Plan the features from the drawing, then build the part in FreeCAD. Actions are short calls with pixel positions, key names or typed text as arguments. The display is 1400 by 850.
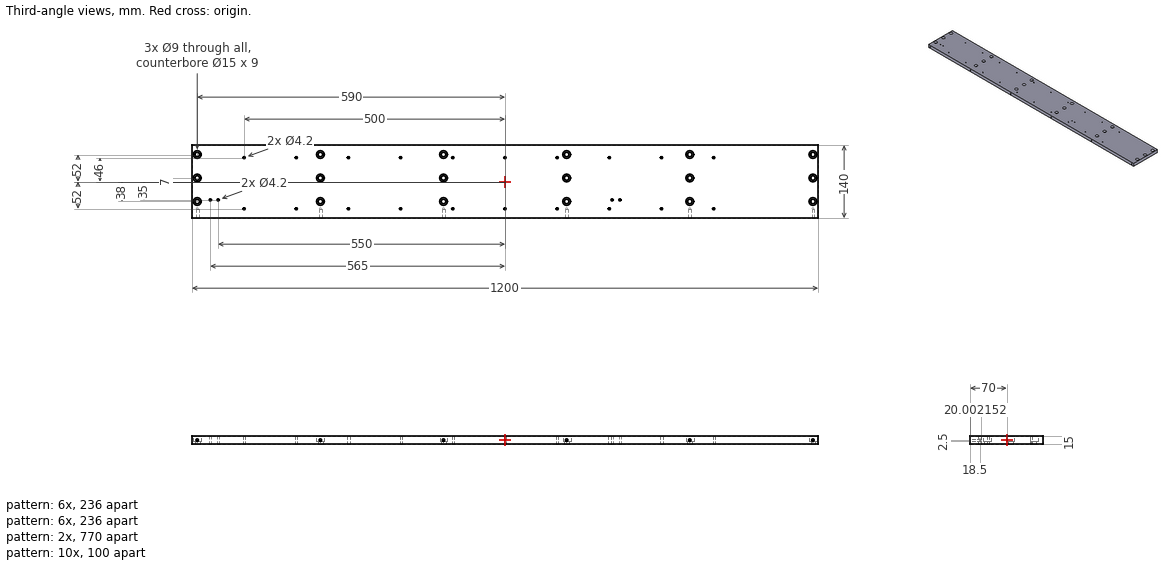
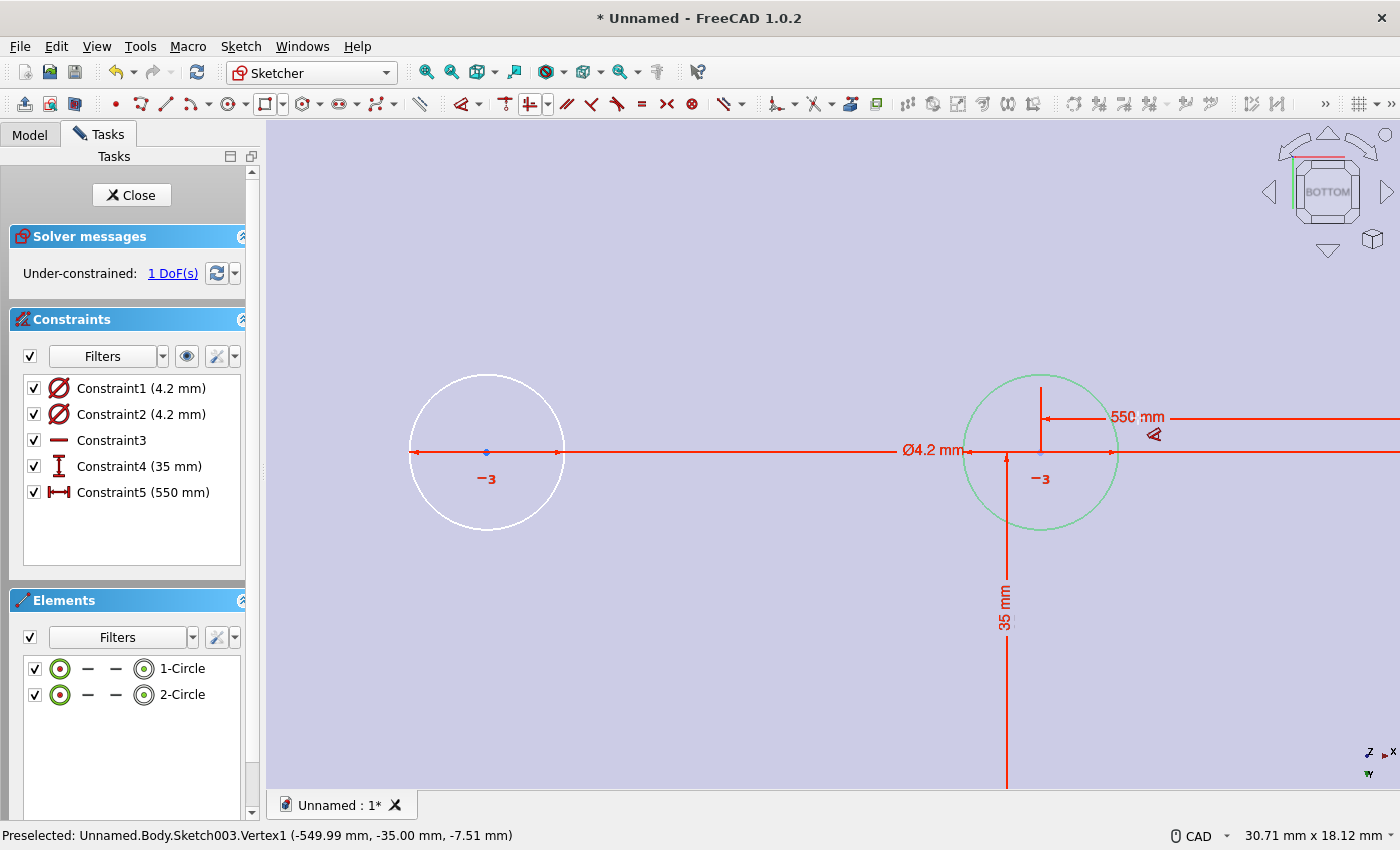
click(487, 452)
click(861, 418)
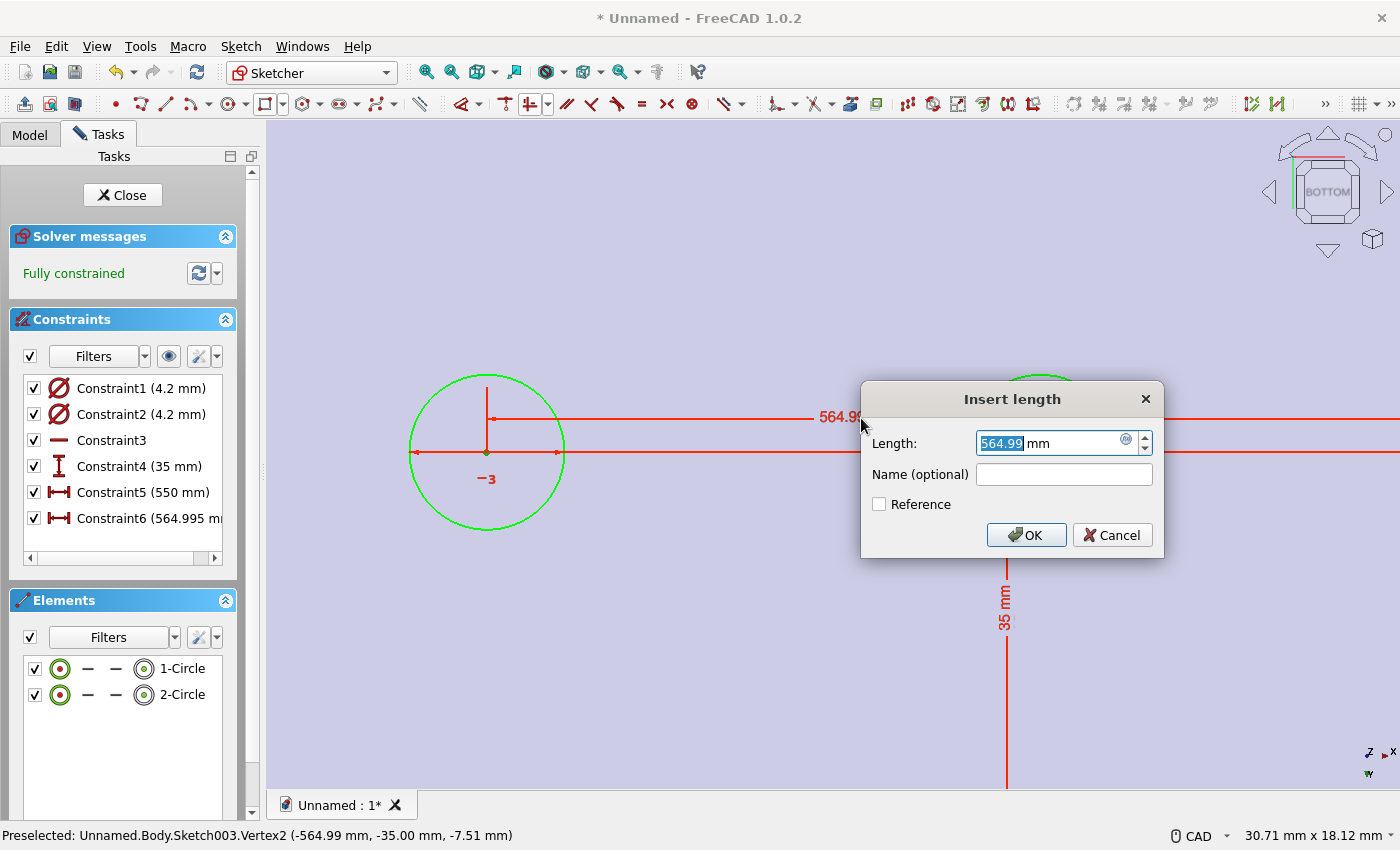
text(565)
key(Return)
key(Escape)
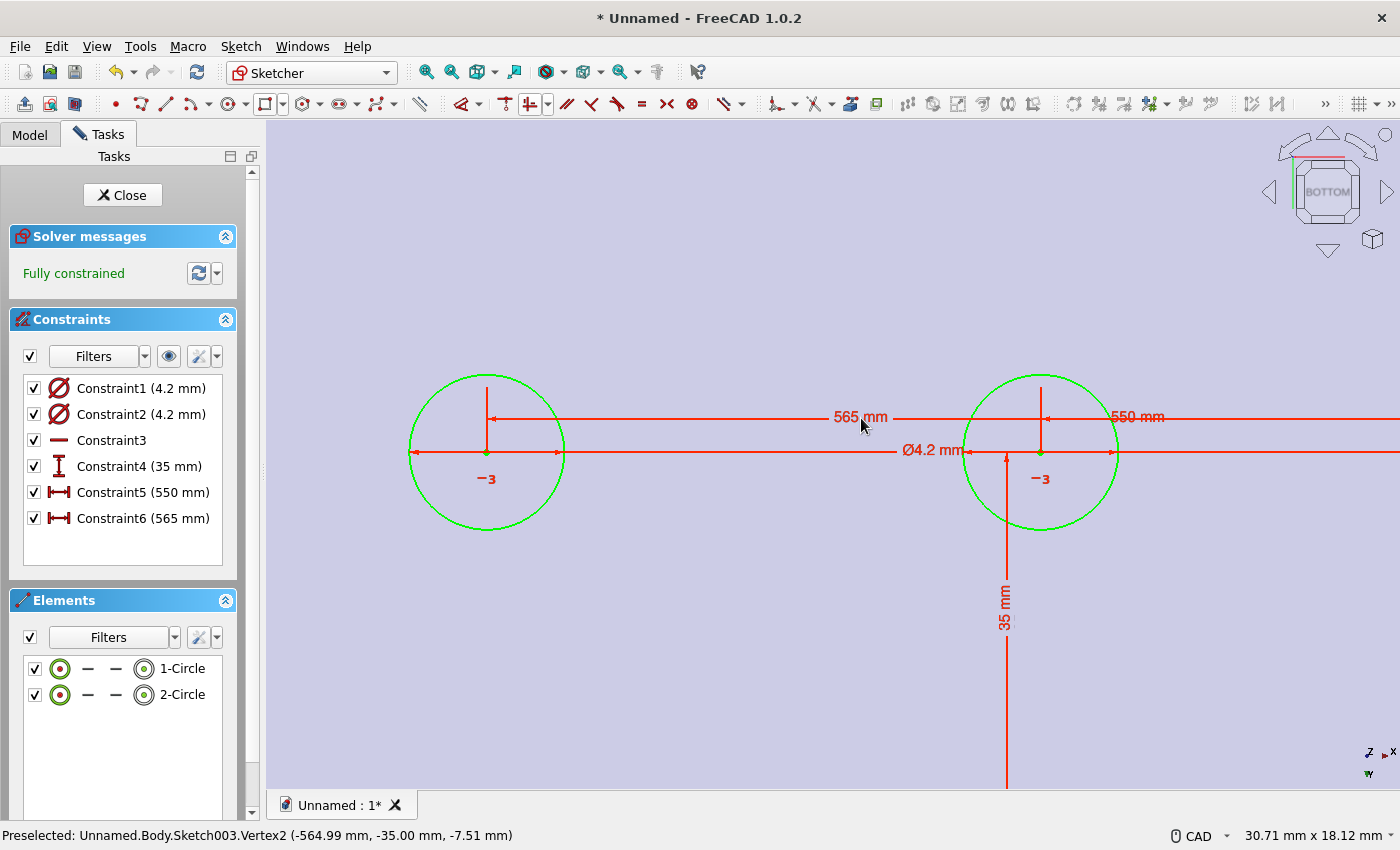
click(123, 195)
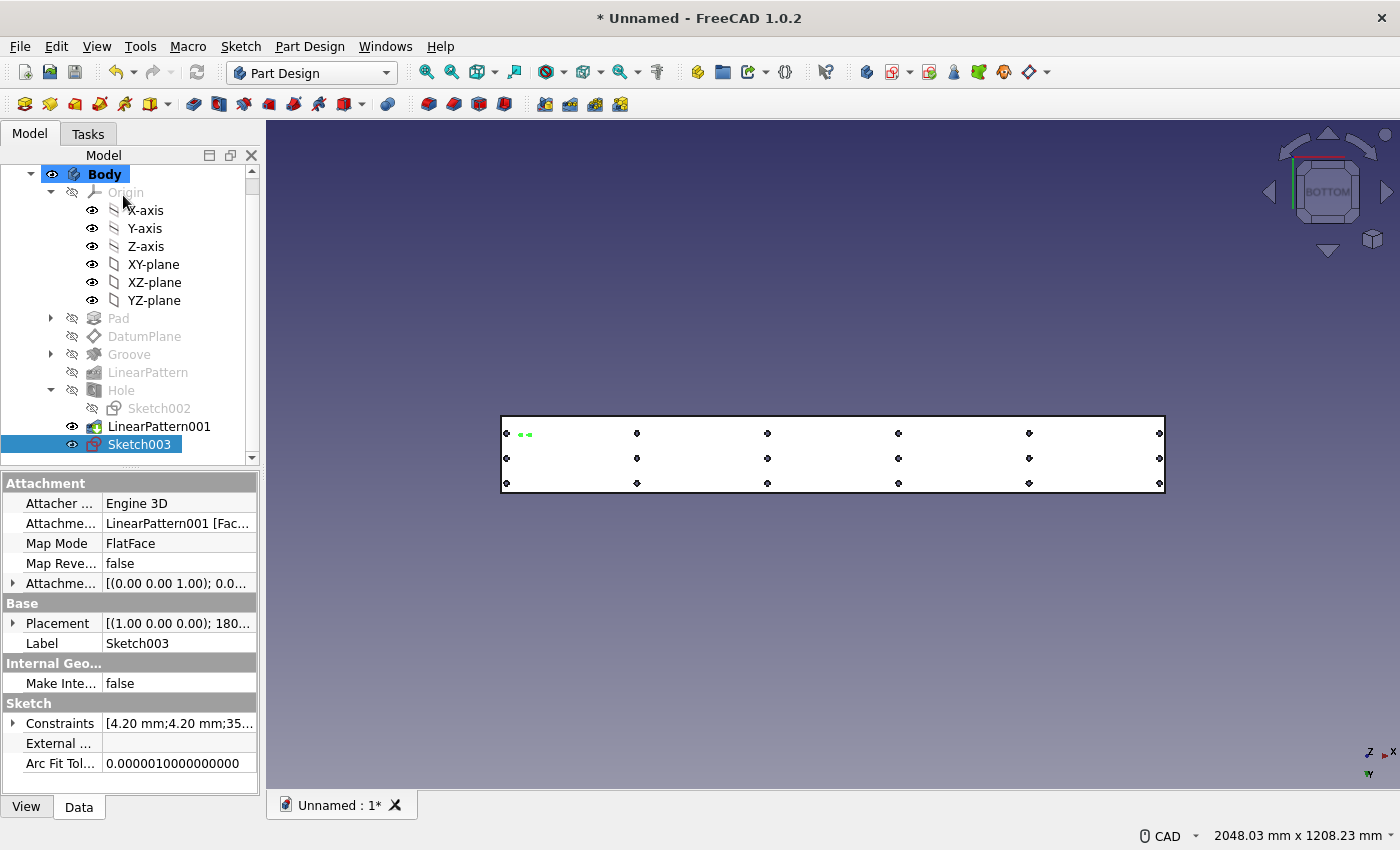
click(194, 104)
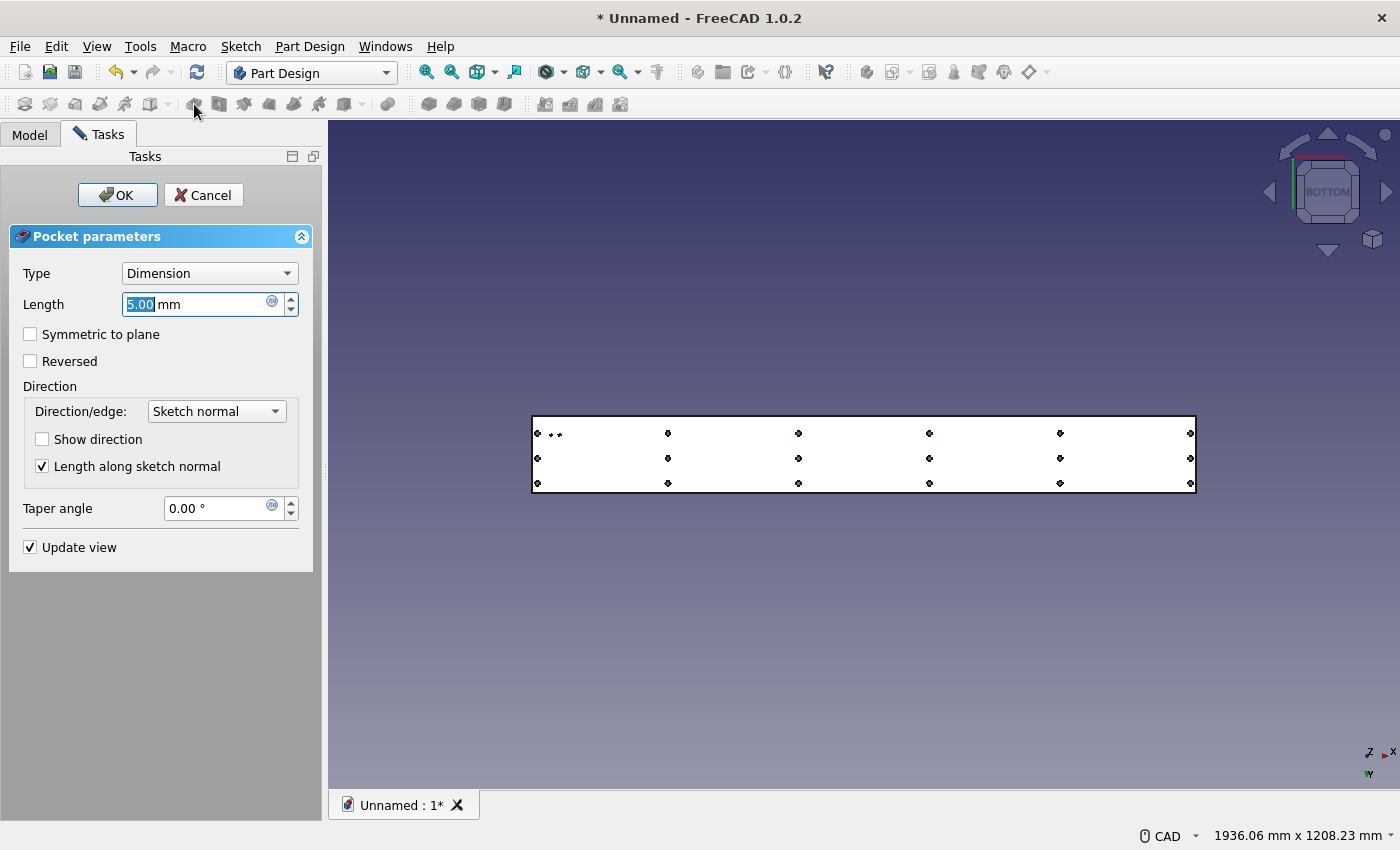
click(210, 274)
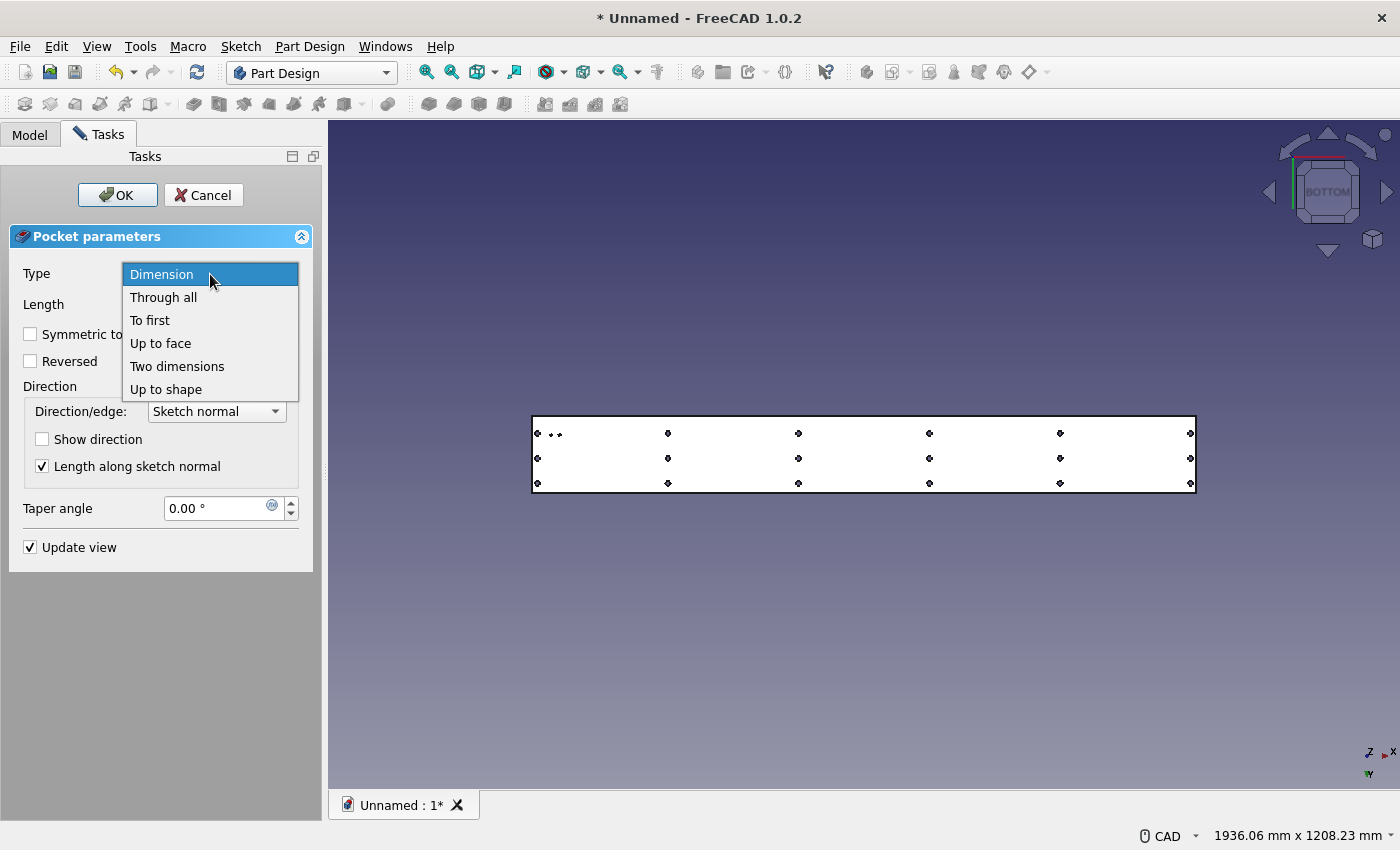
click(208, 298)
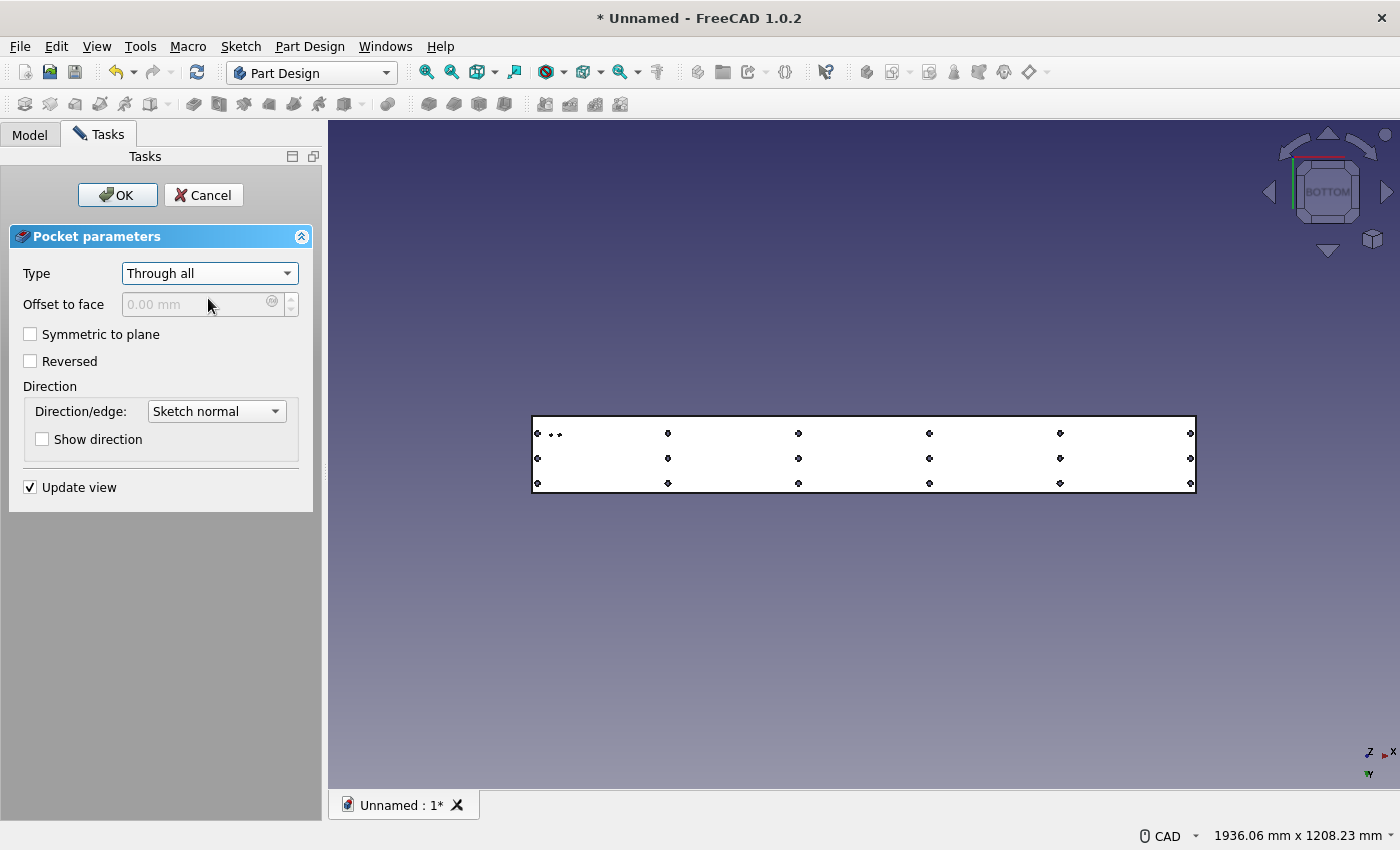
click(118, 195)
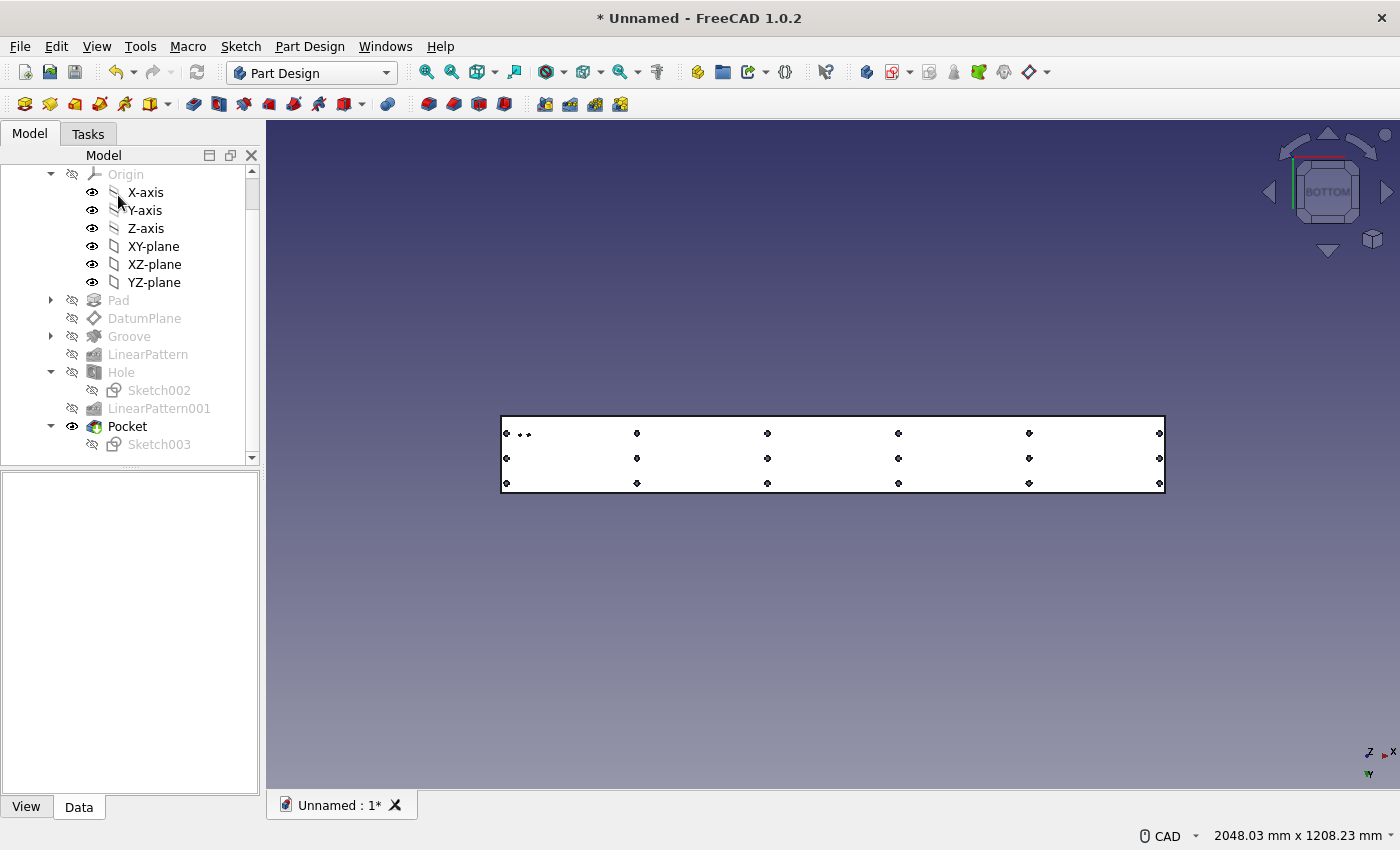
click(117, 426)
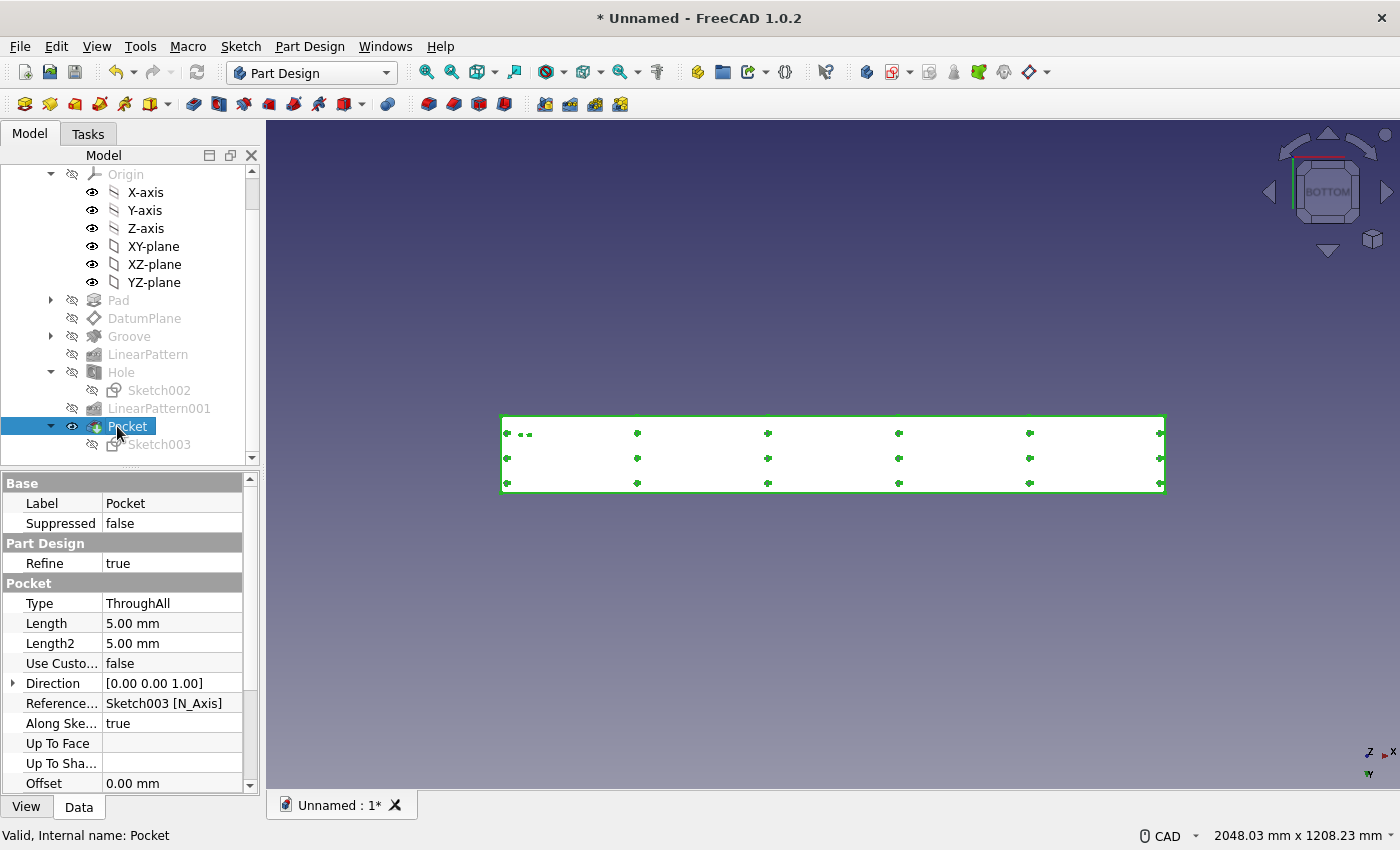
click(570, 104)